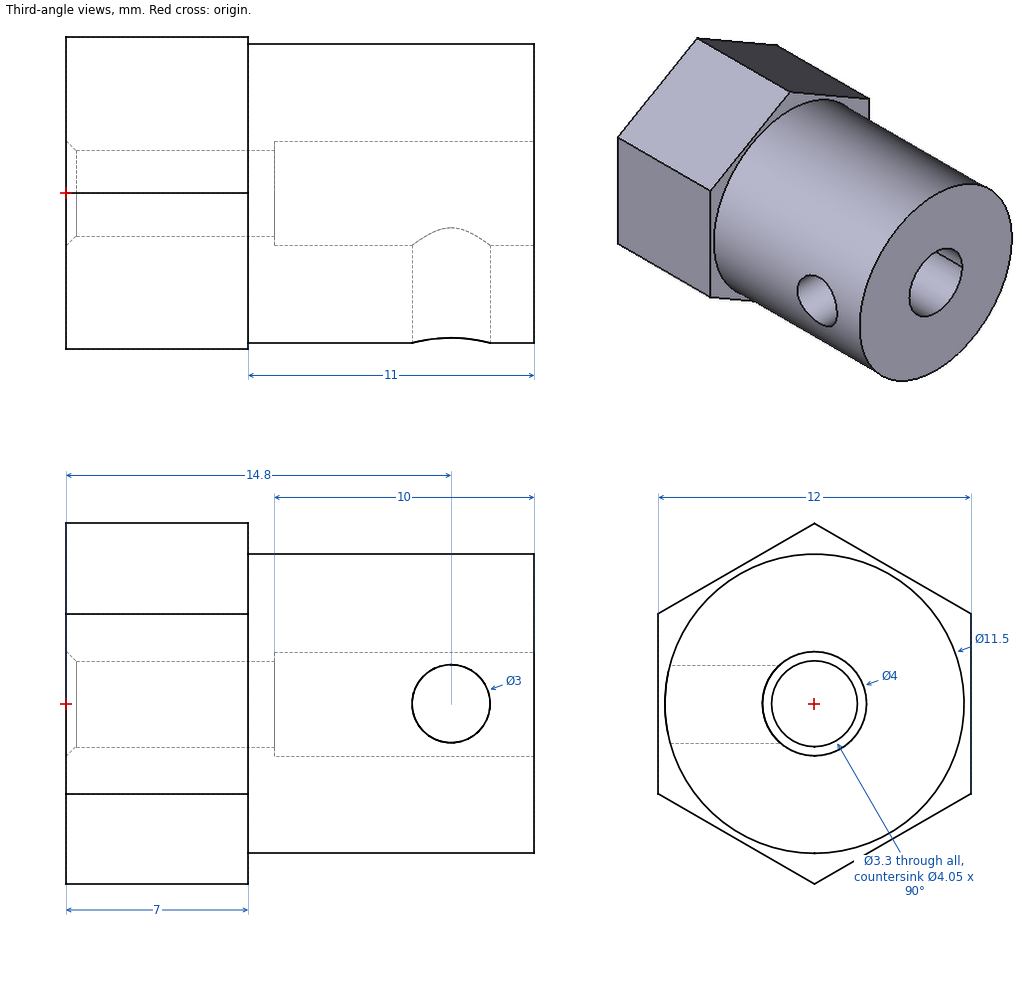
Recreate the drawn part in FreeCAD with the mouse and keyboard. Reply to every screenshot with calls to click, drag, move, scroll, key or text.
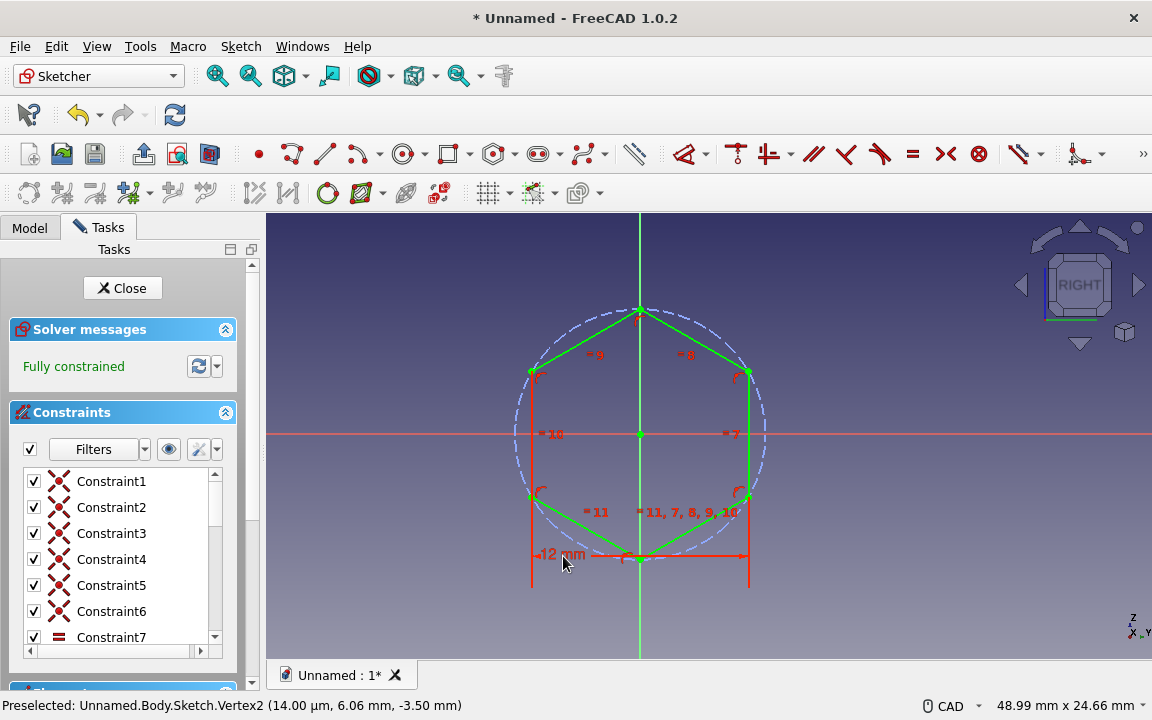
click(123, 288)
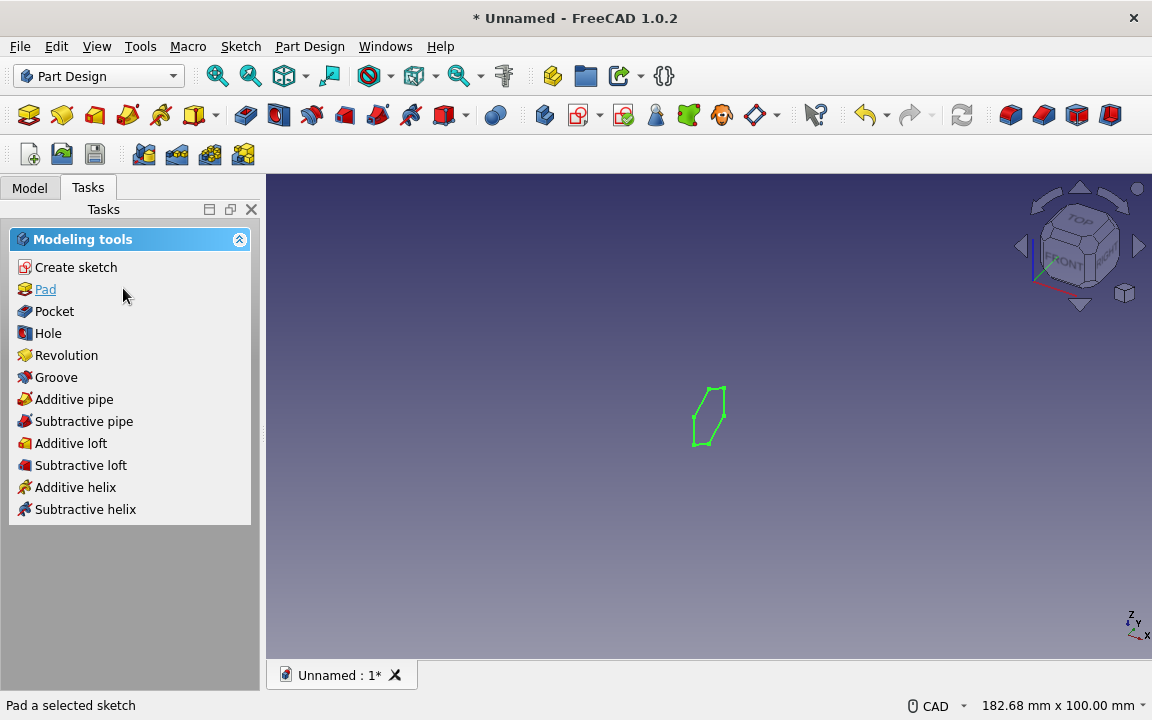
click(29, 116)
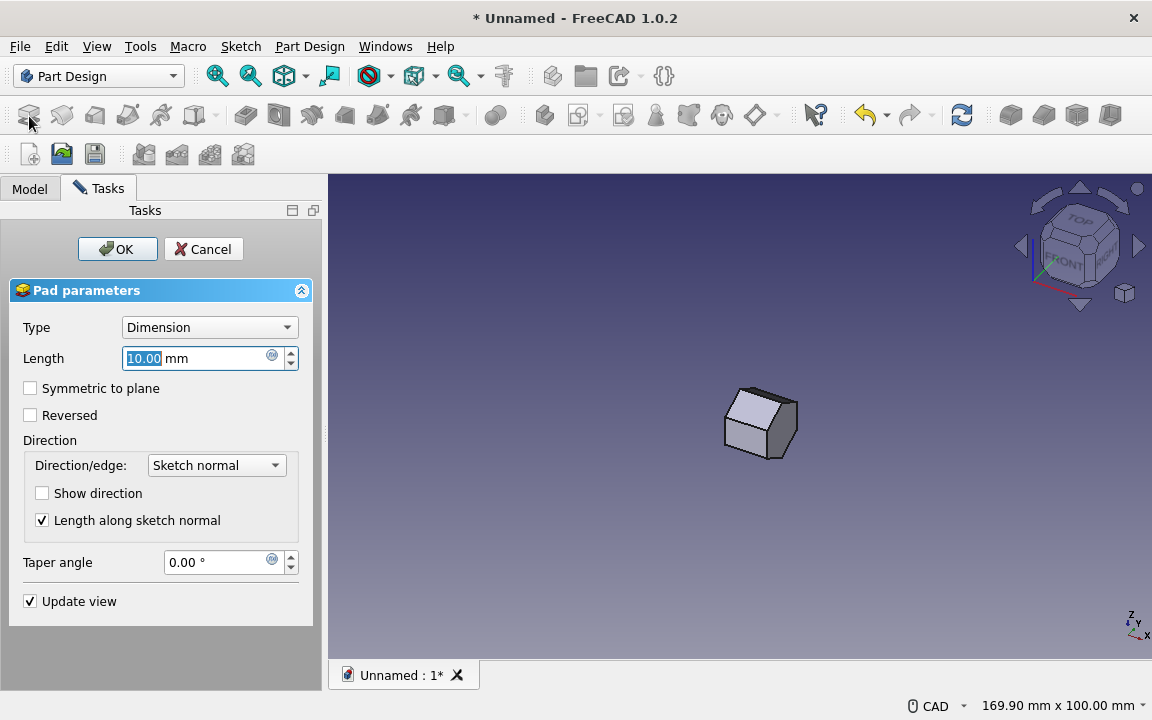
text(7)
key(Tab)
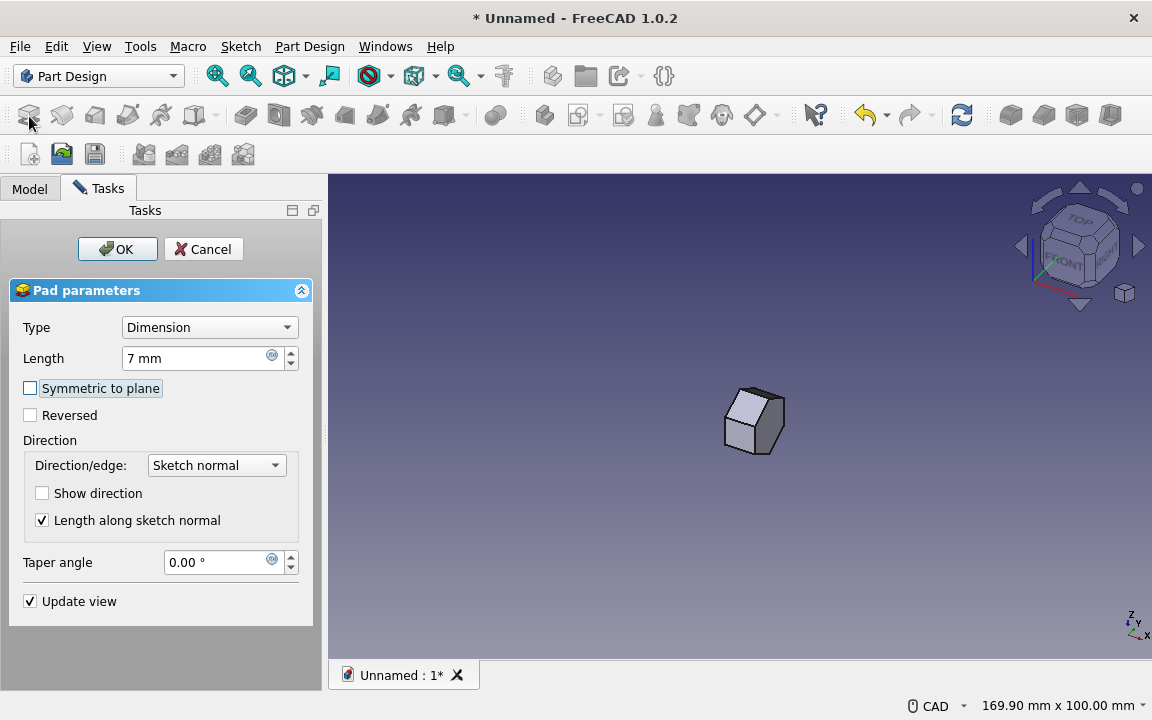
click(118, 249)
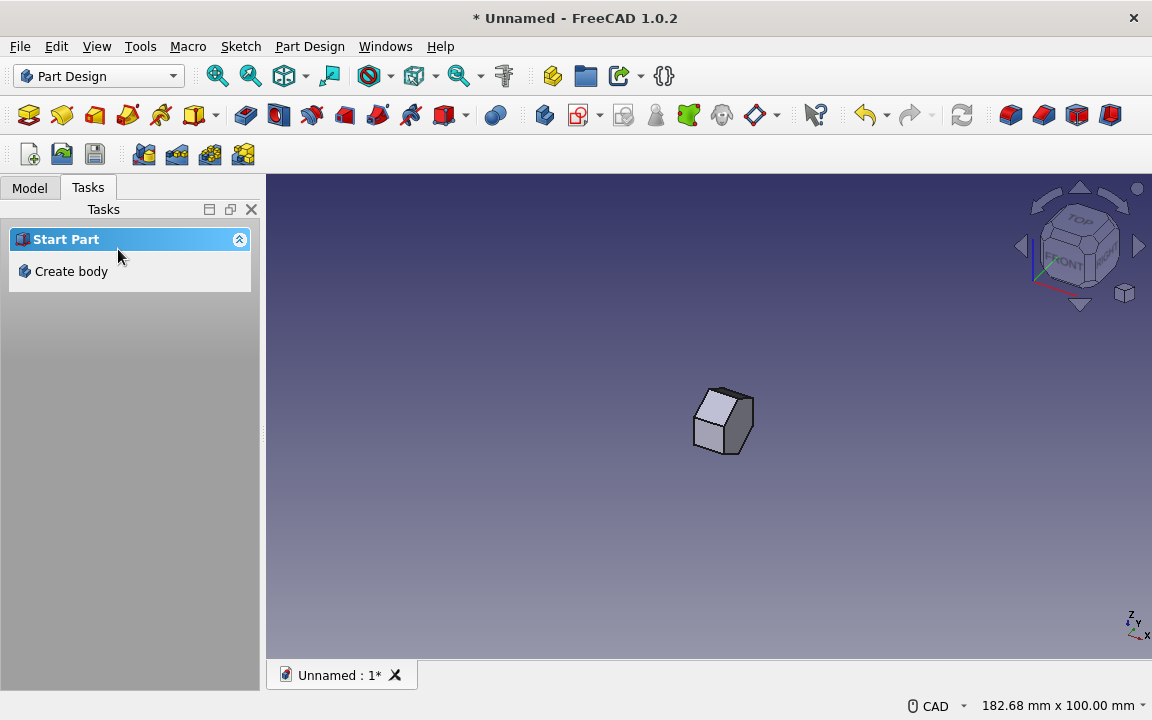
click(218, 76)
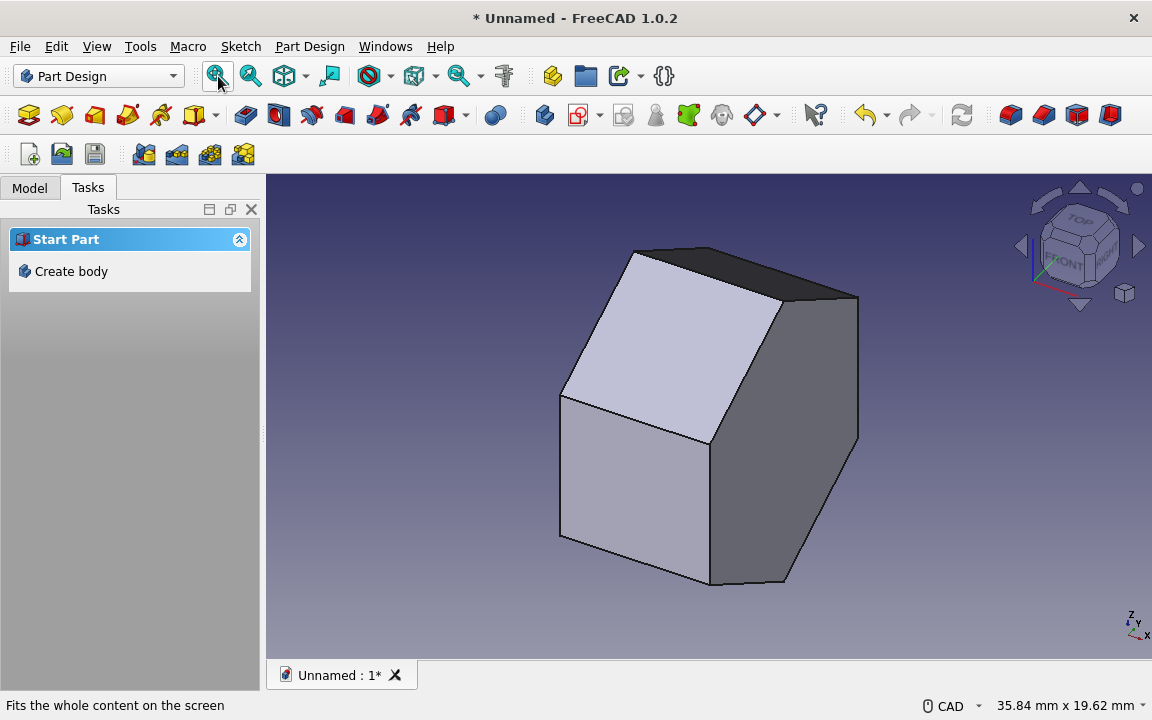
click(784, 440)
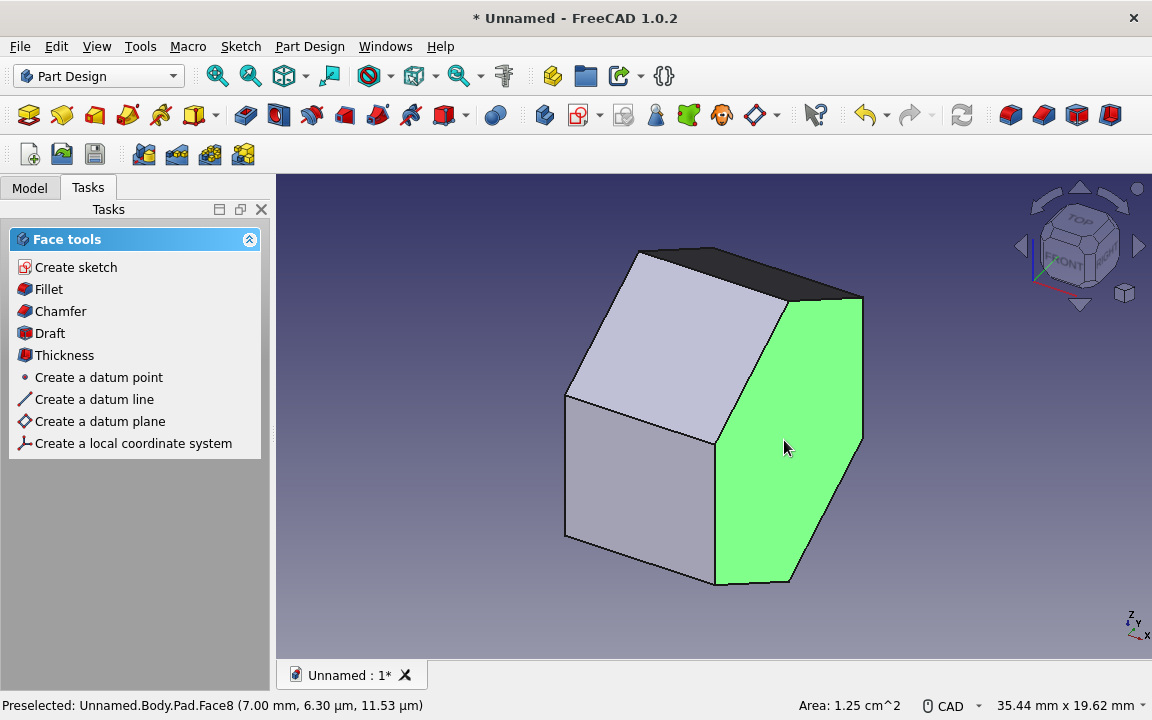
click(578, 116)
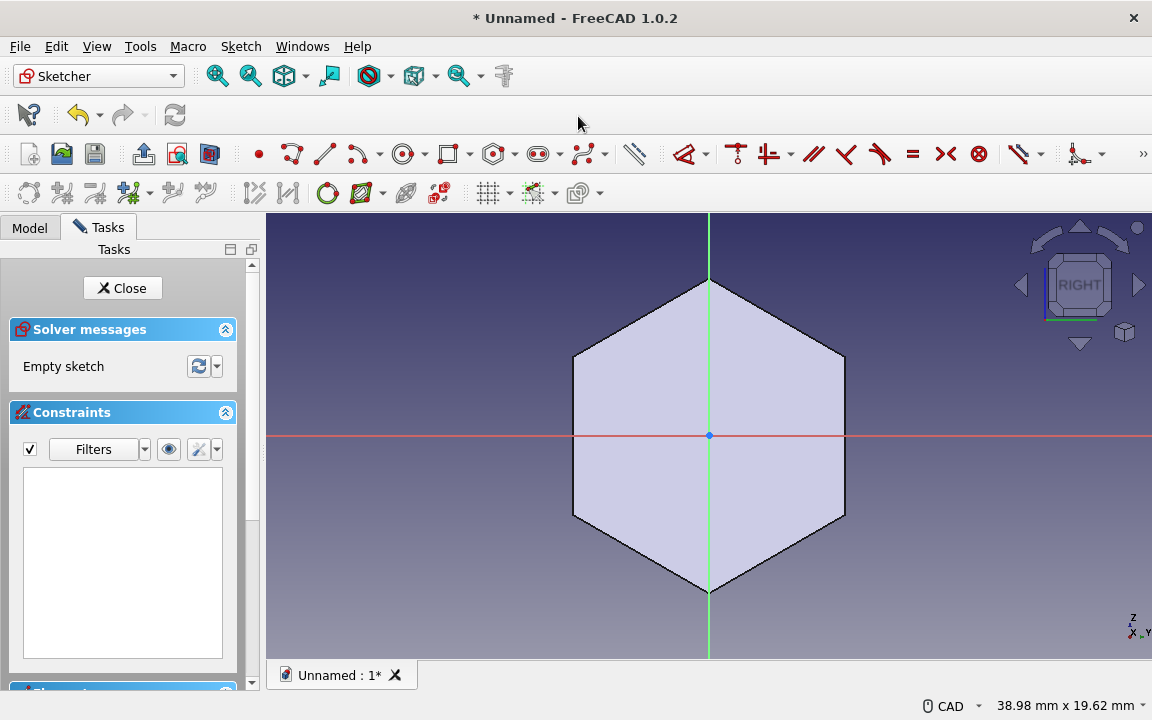
key(g)
key(c)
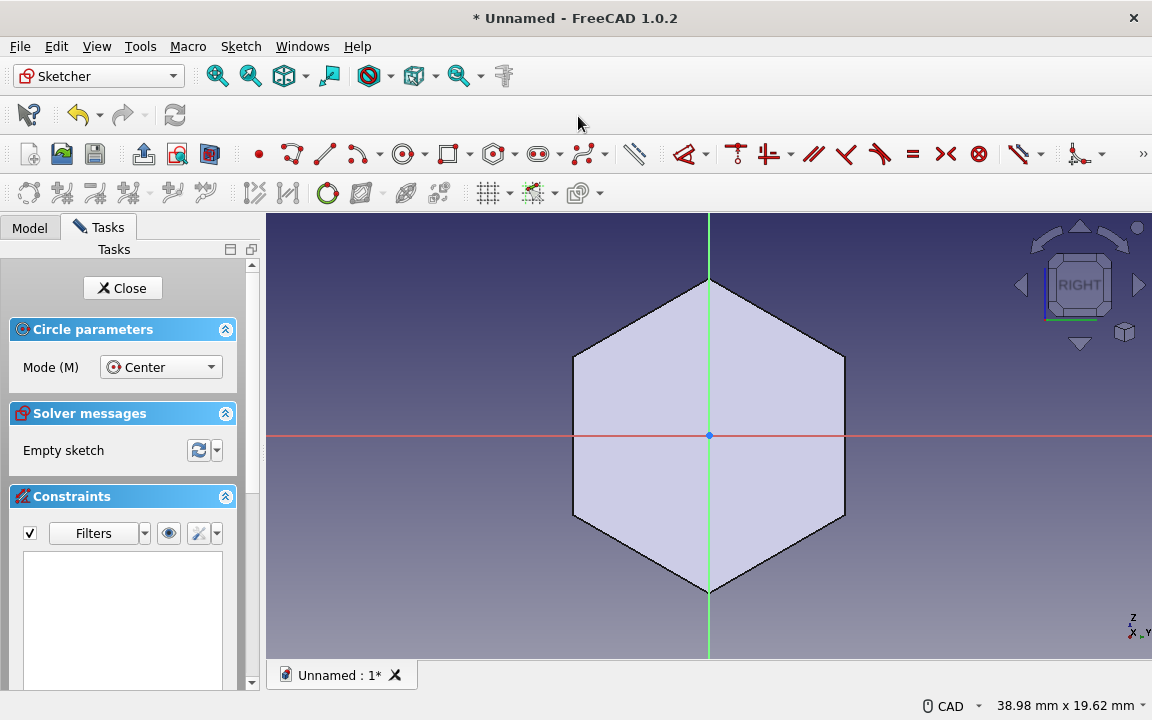
click(709, 436)
move(801, 344)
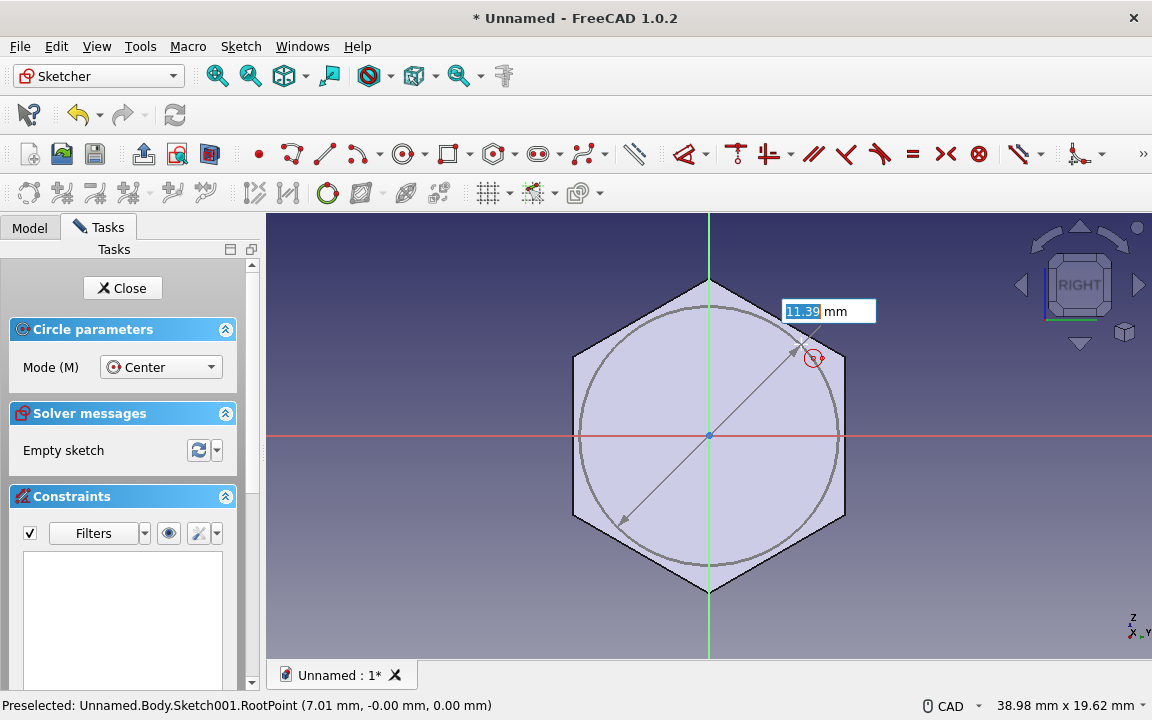
text(11.5)
key(Return)
key(Escape)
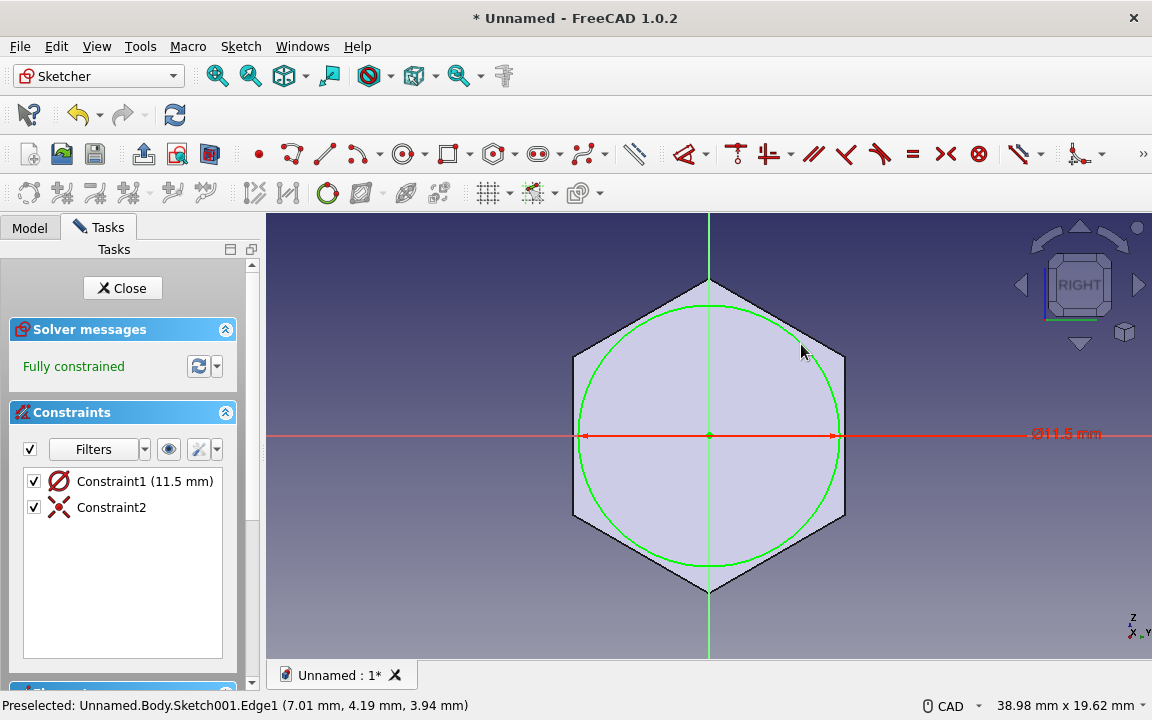
click(123, 288)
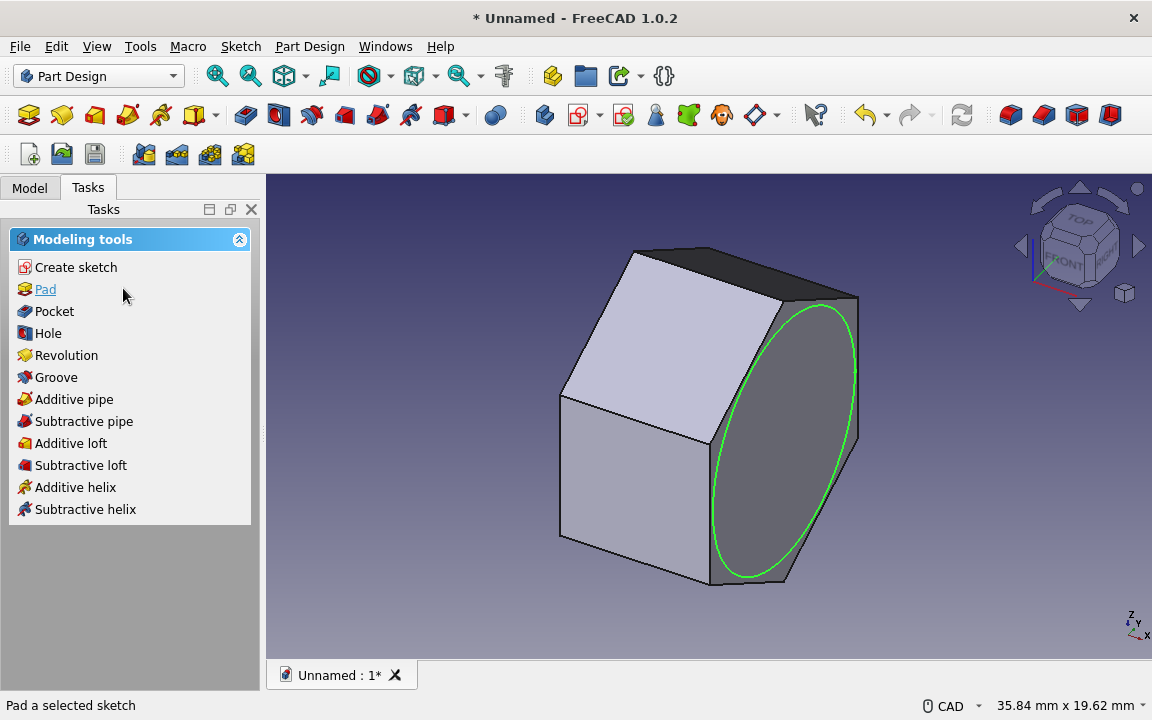
click(29, 116)